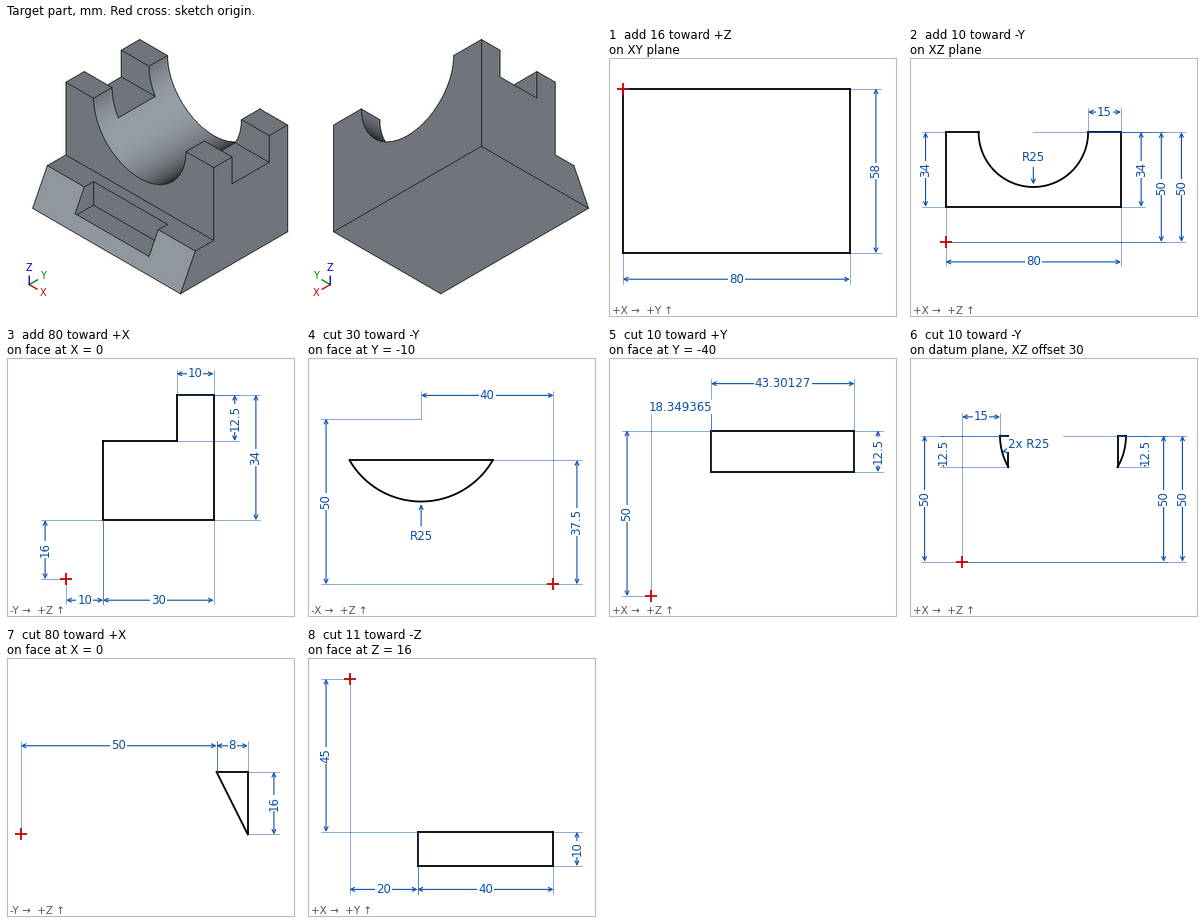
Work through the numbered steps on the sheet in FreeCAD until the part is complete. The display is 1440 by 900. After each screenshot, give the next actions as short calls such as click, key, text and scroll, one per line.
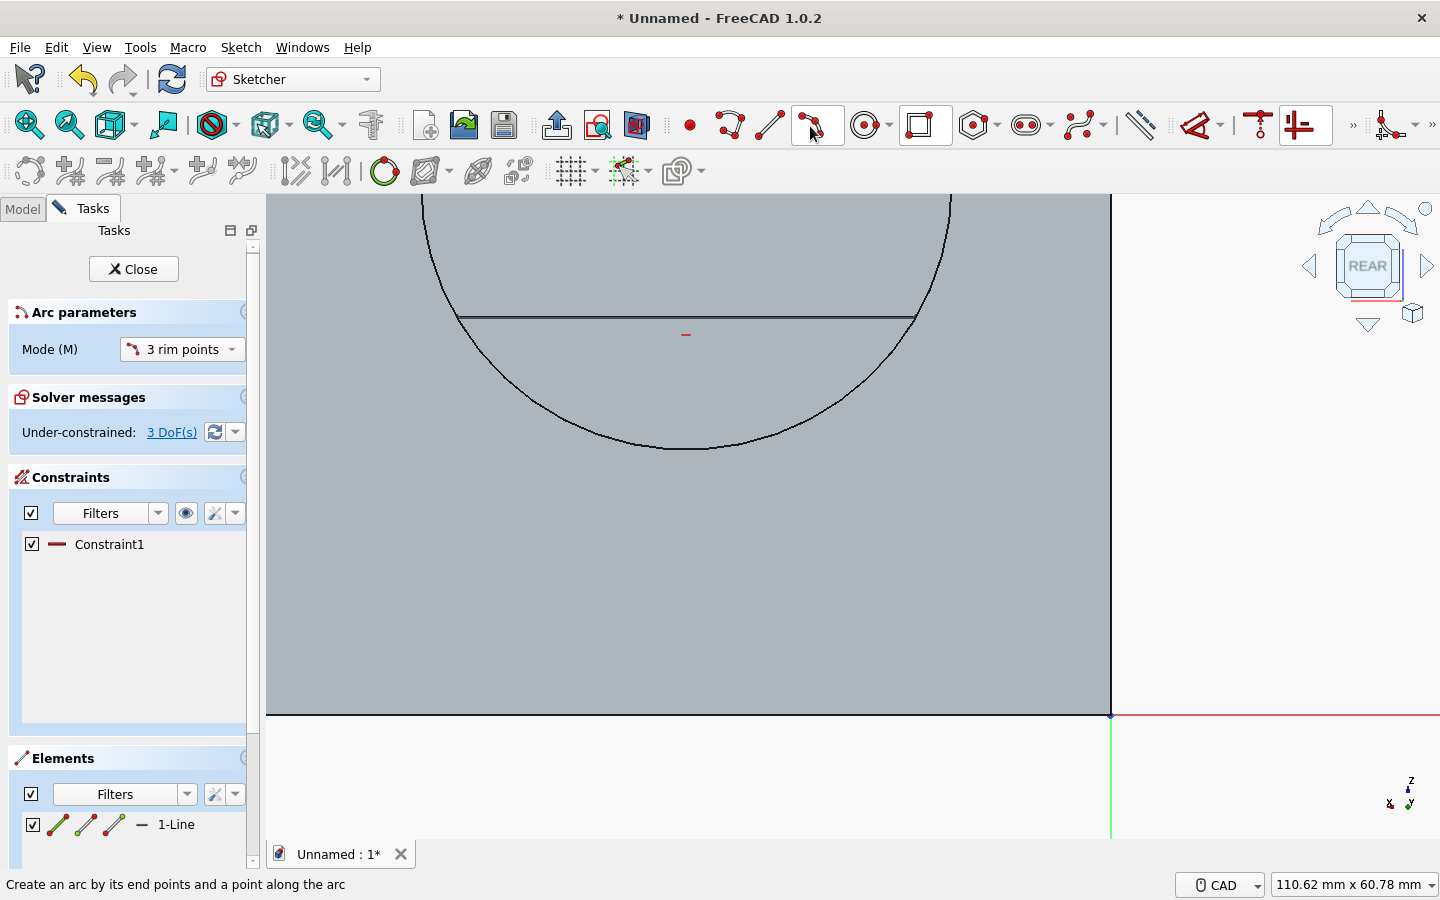
click(457, 318)
click(916, 318)
click(686, 450)
key(Escape)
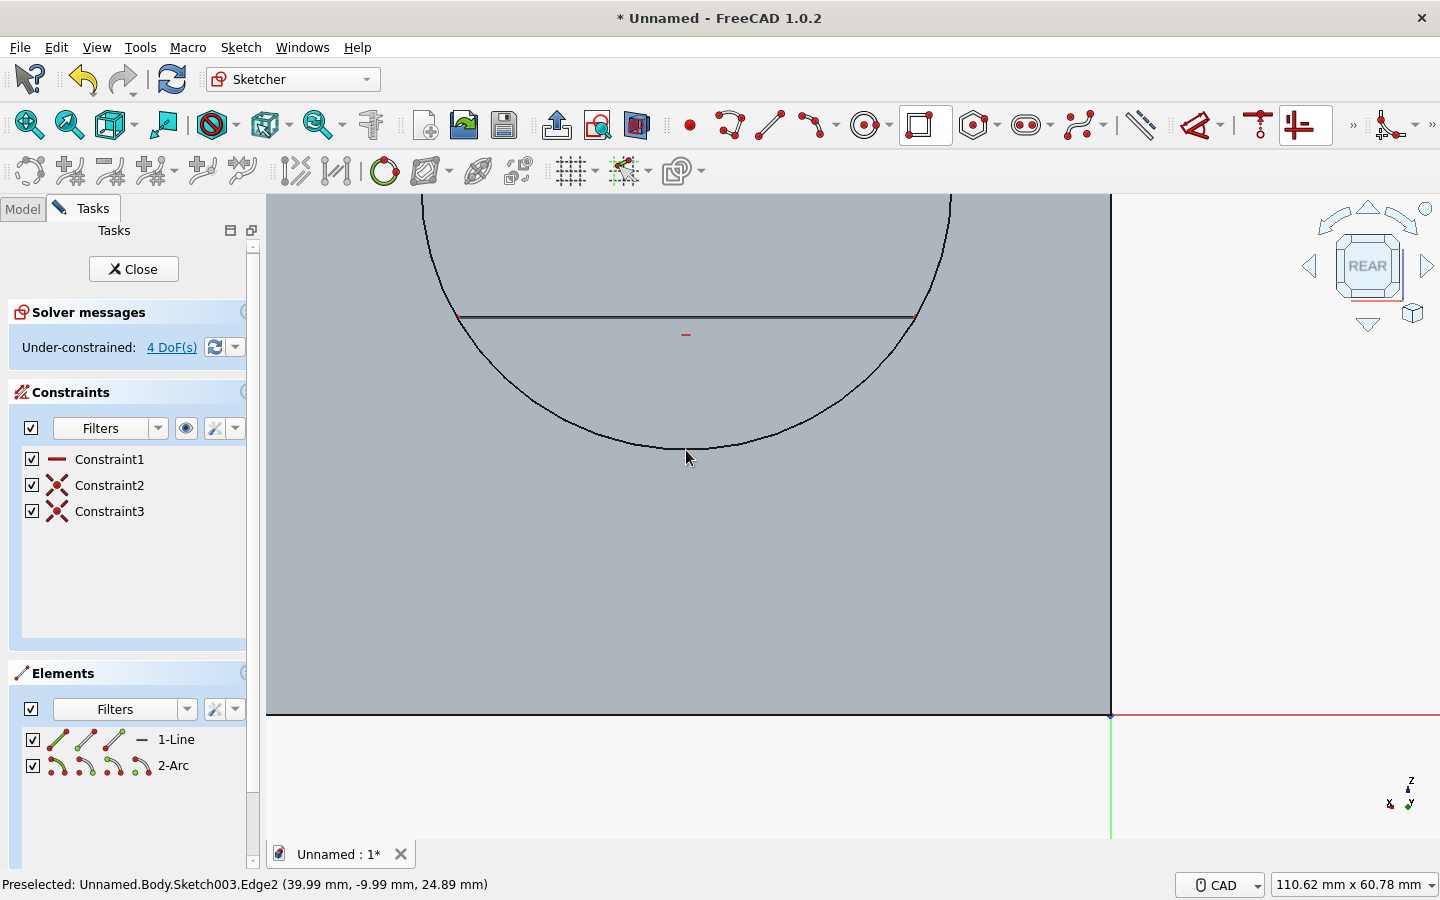
click(1196, 126)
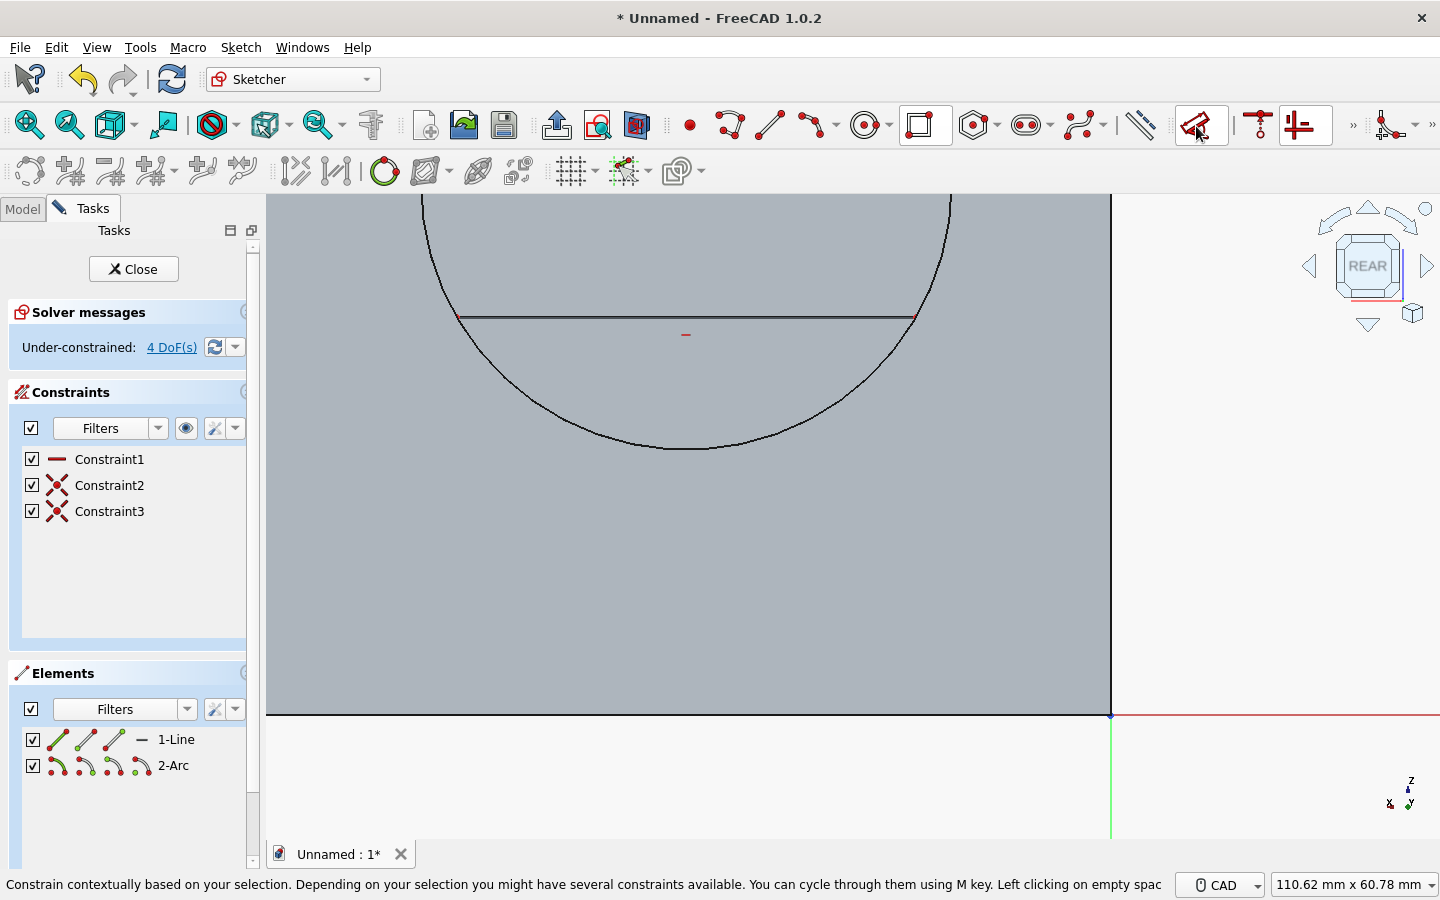
click(579, 428)
click(566, 457)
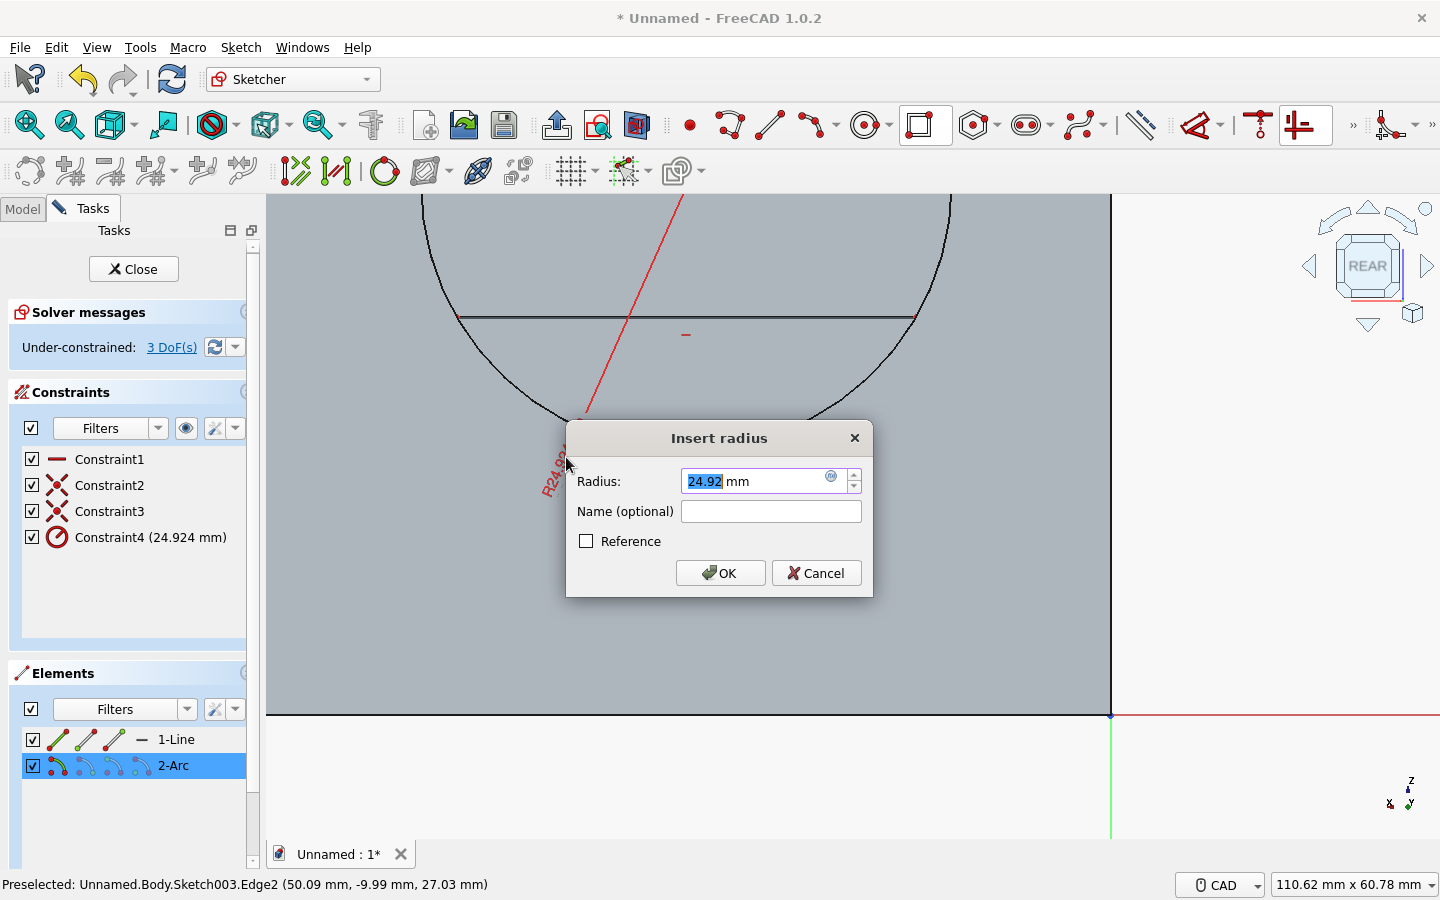
text(25)
key(Return)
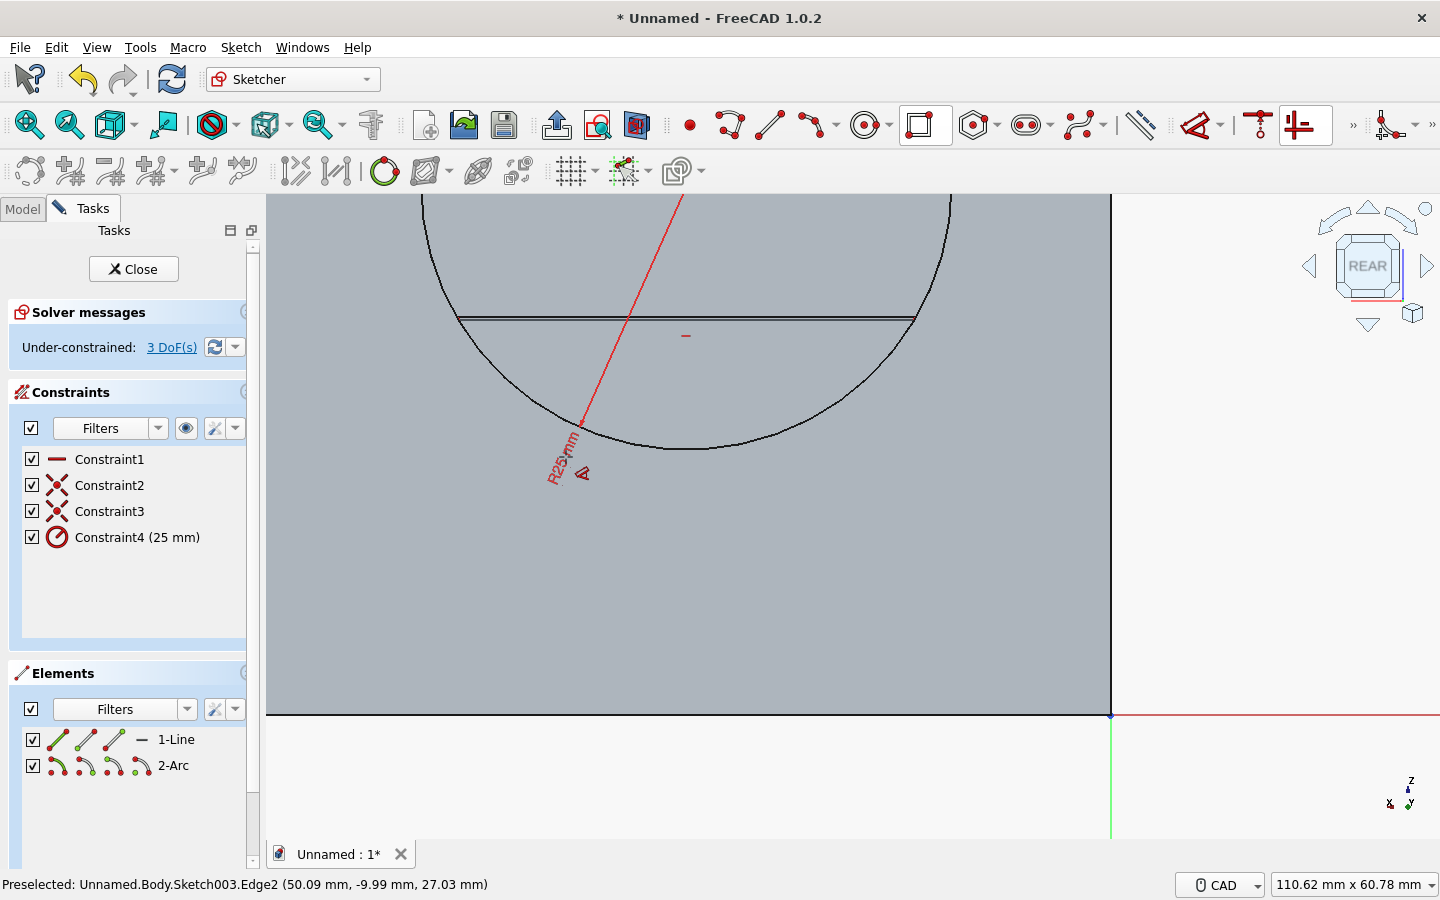
scroll(788, 811, down, 1)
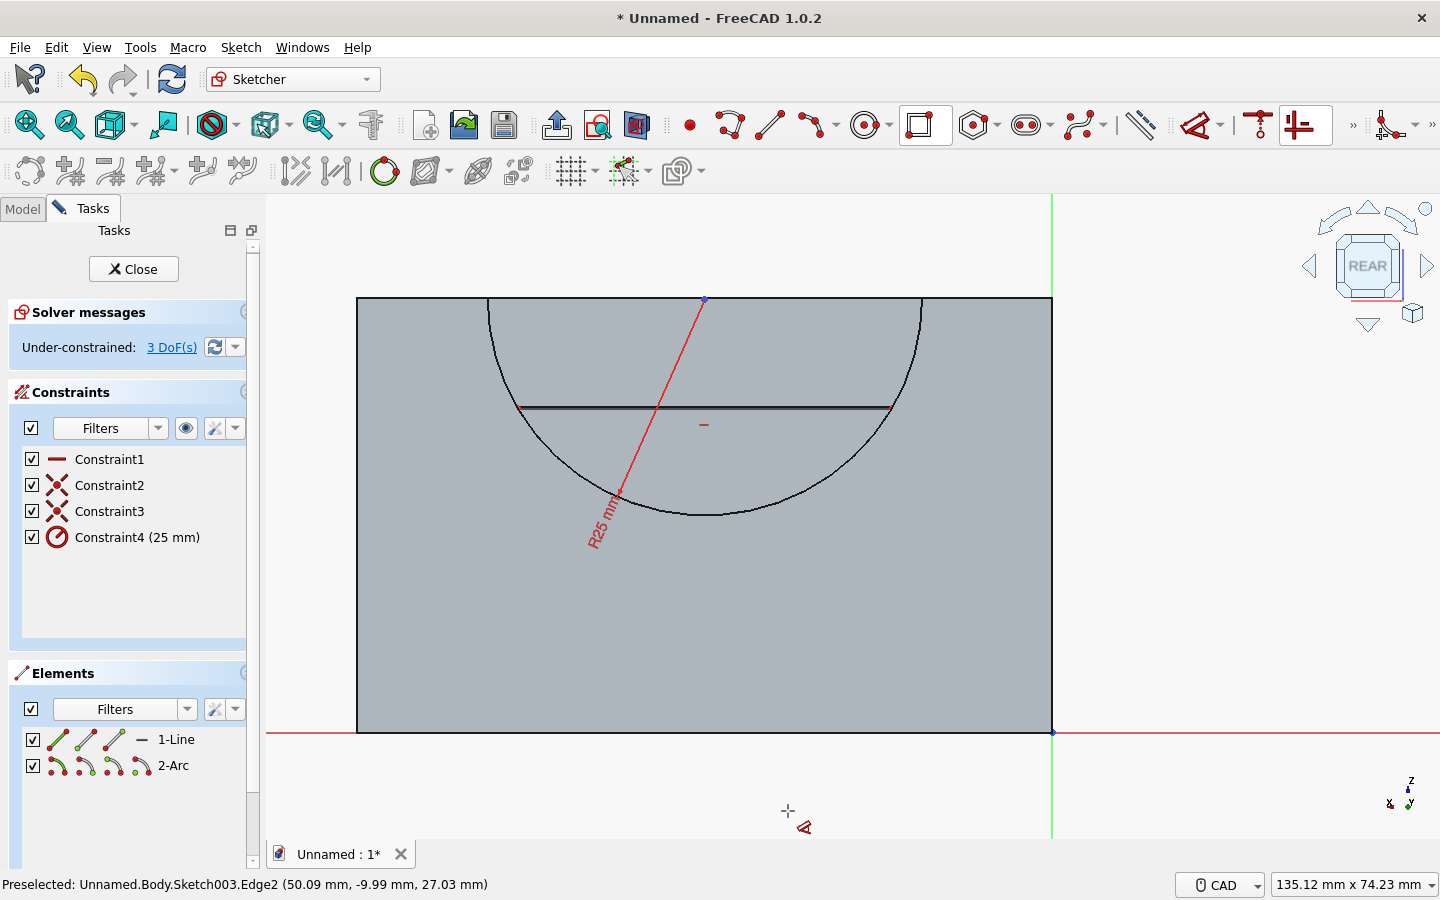
click(705, 300)
click(879, 266)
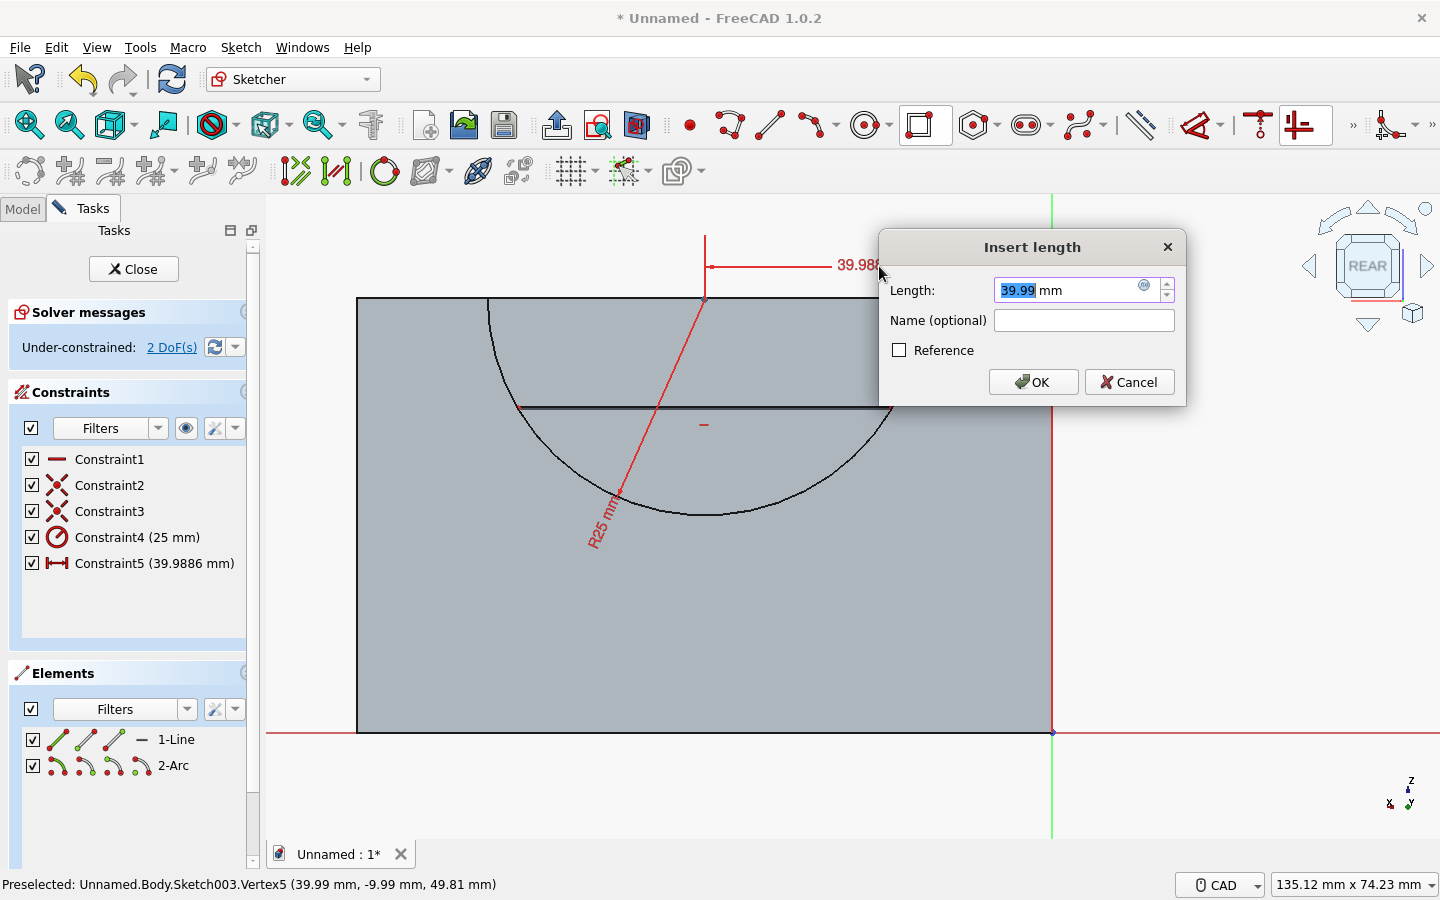
text(40)
key(Return)